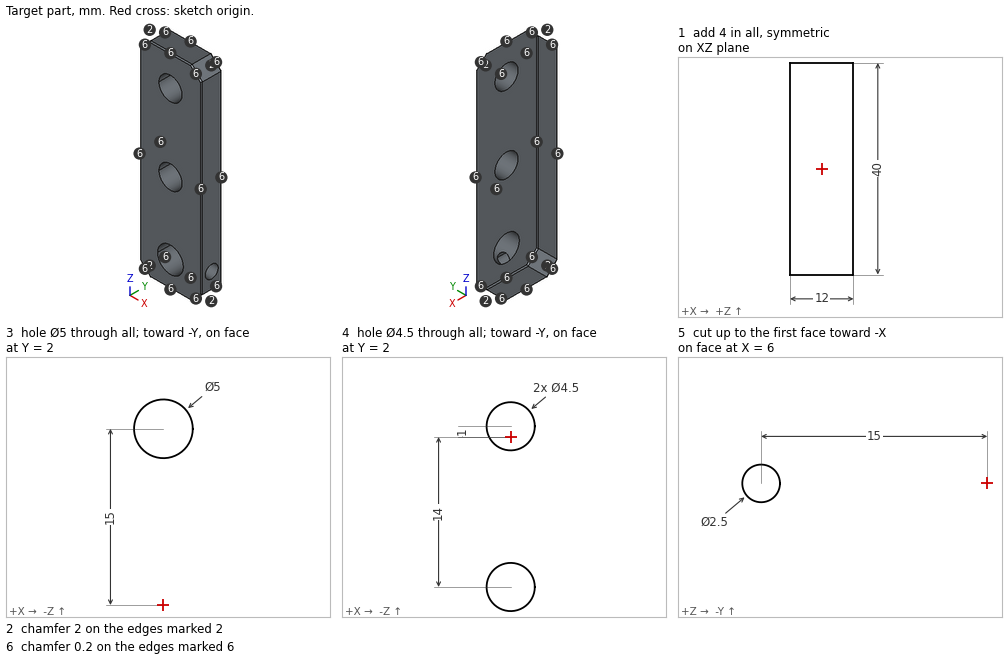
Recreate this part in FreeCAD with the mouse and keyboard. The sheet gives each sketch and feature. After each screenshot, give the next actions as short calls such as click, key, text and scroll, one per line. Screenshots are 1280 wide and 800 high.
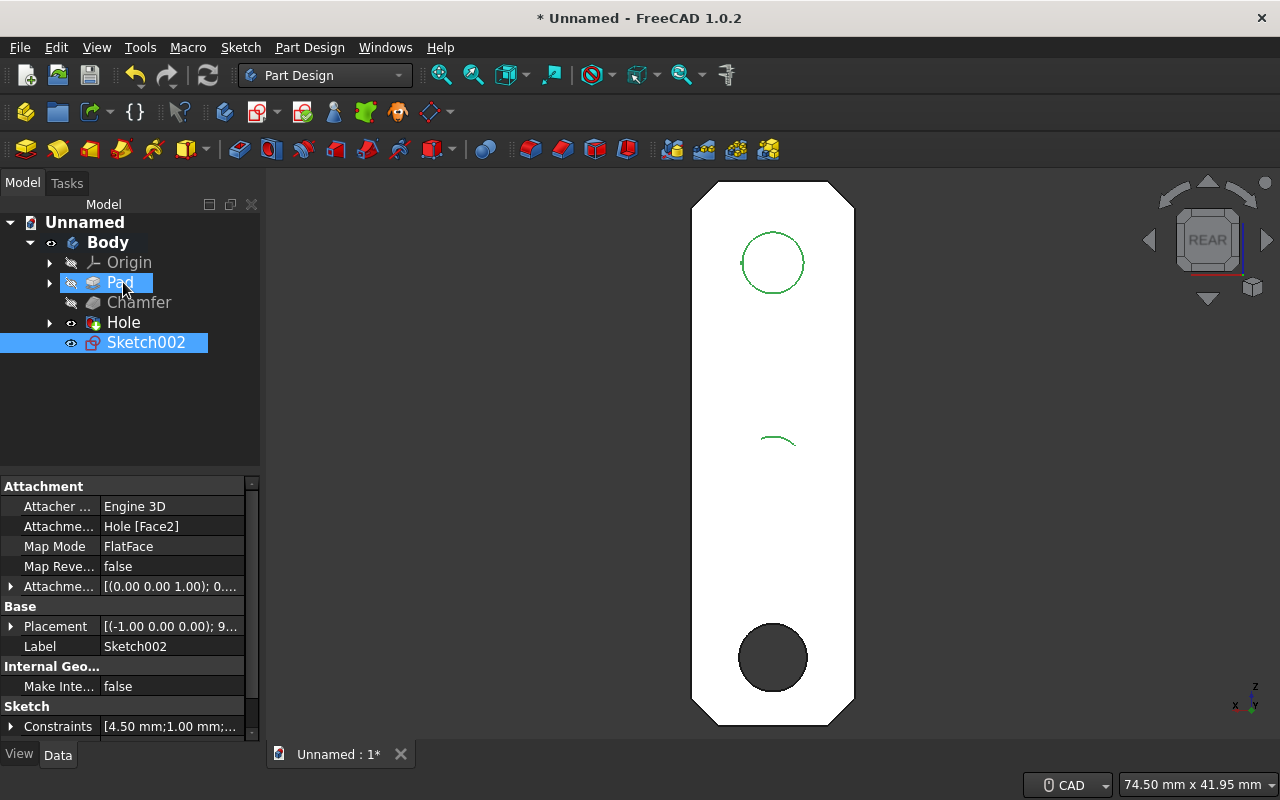
click(272, 150)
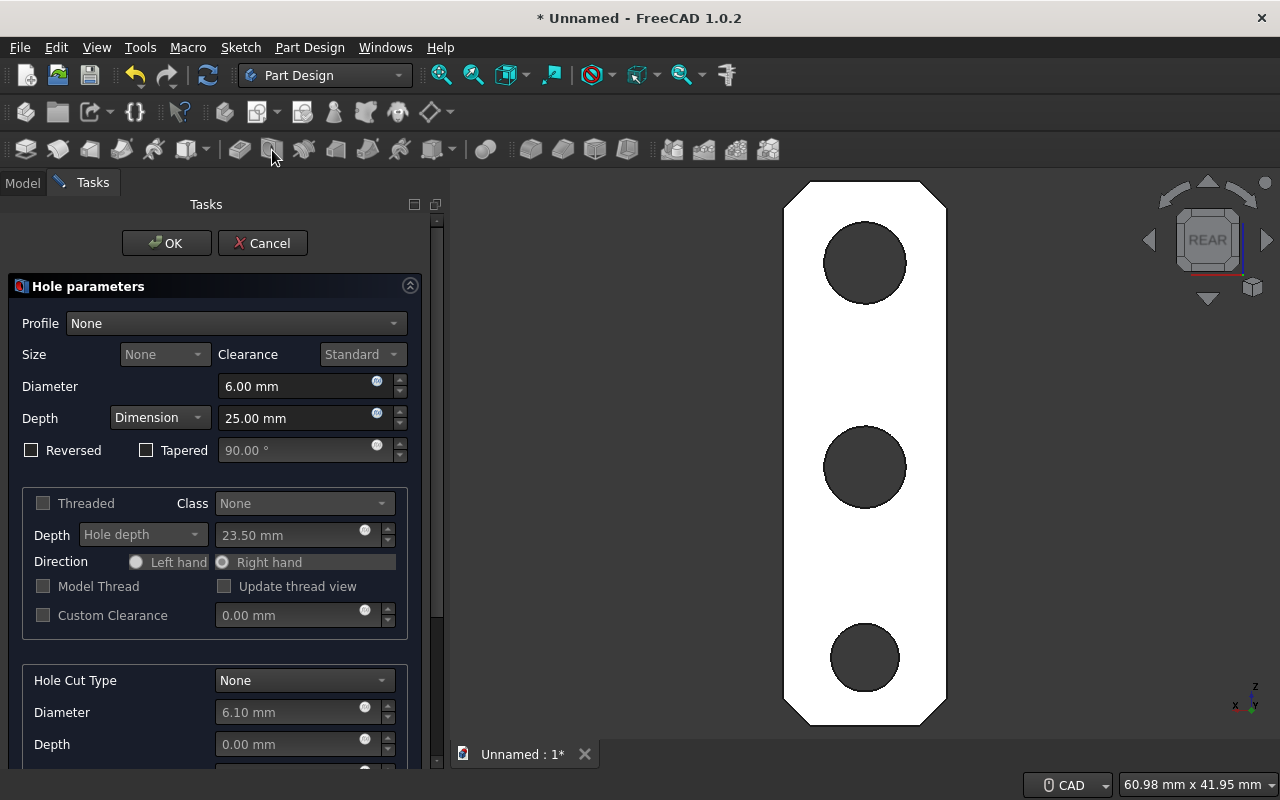
triple_click(305, 386)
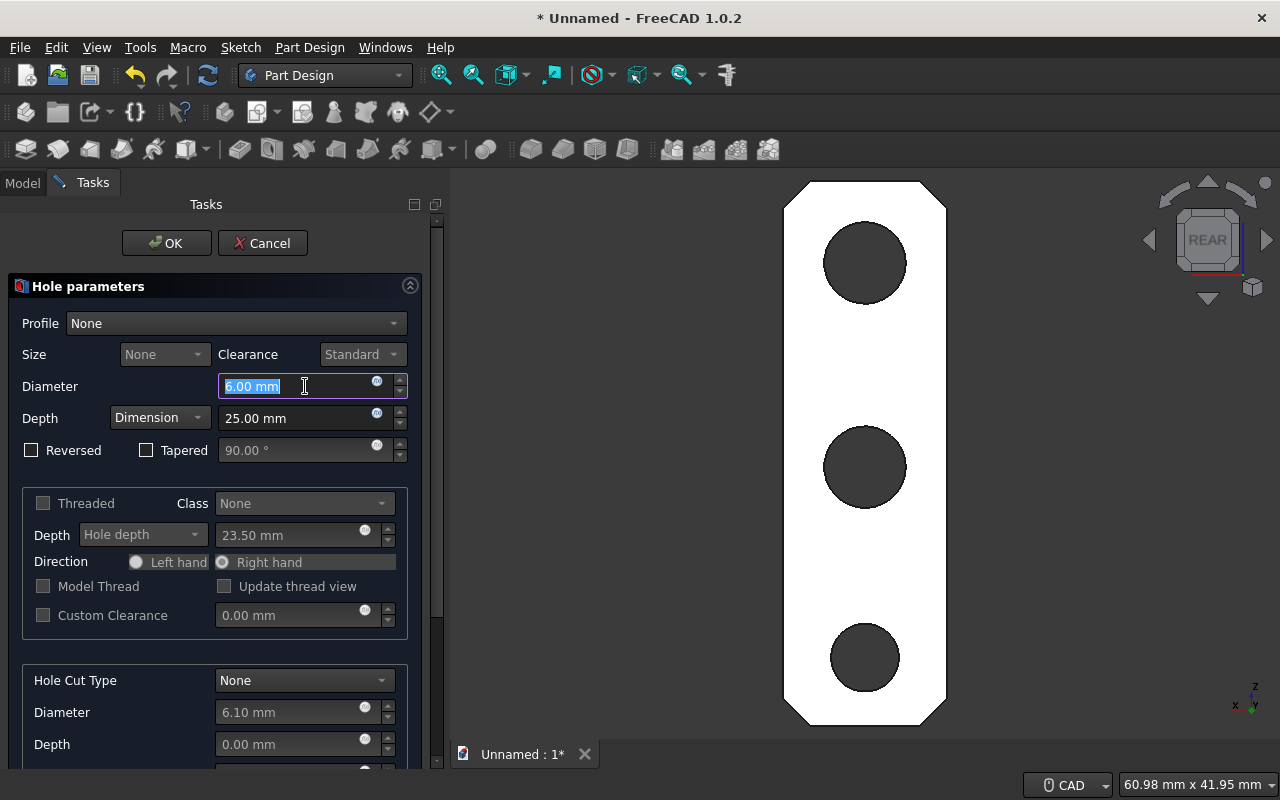
text(4.5)
key(Tab)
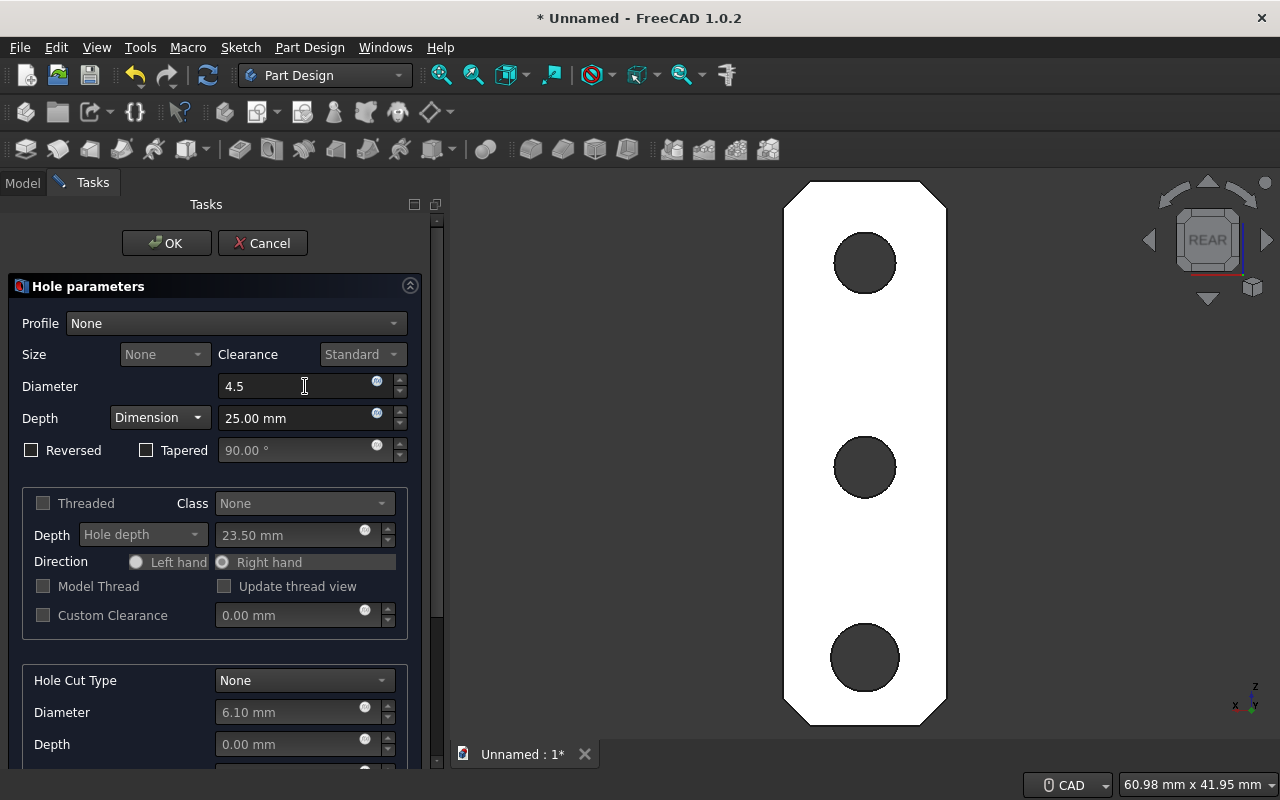
click(161, 418)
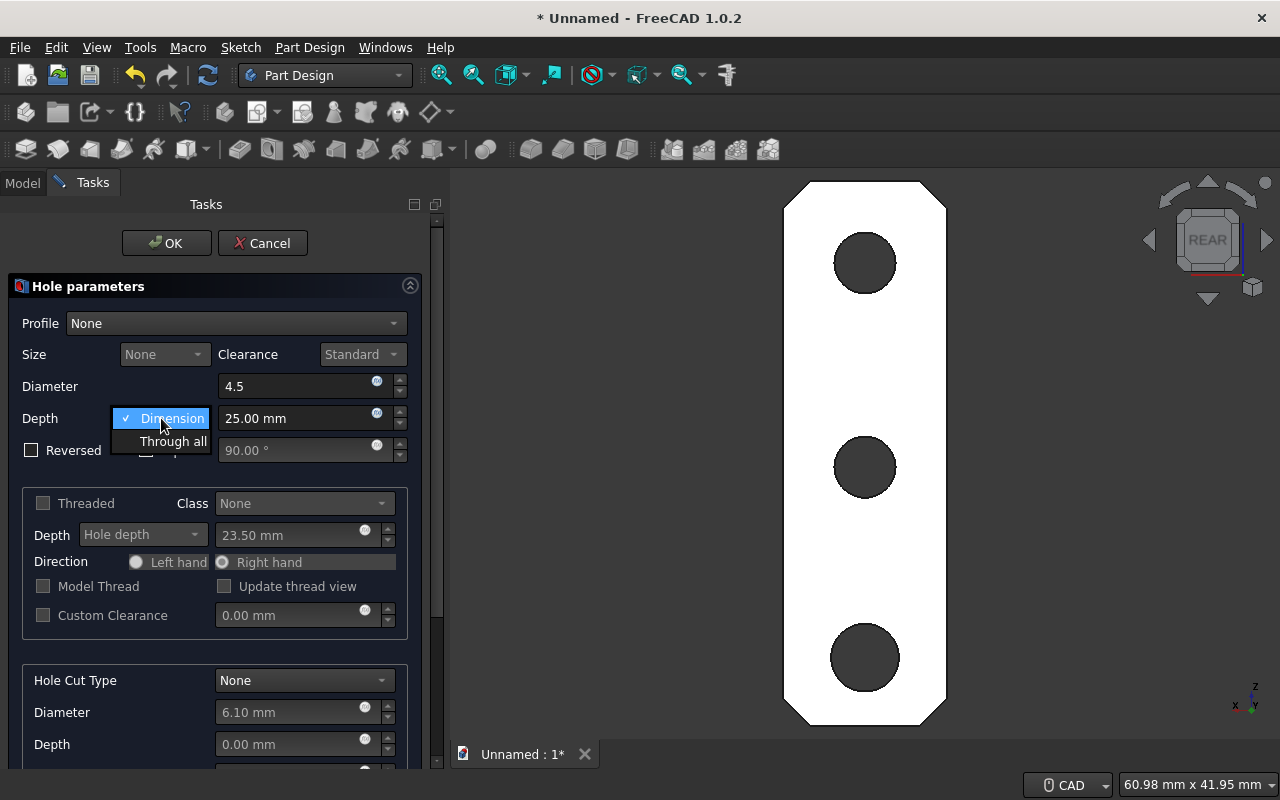
click(160, 442)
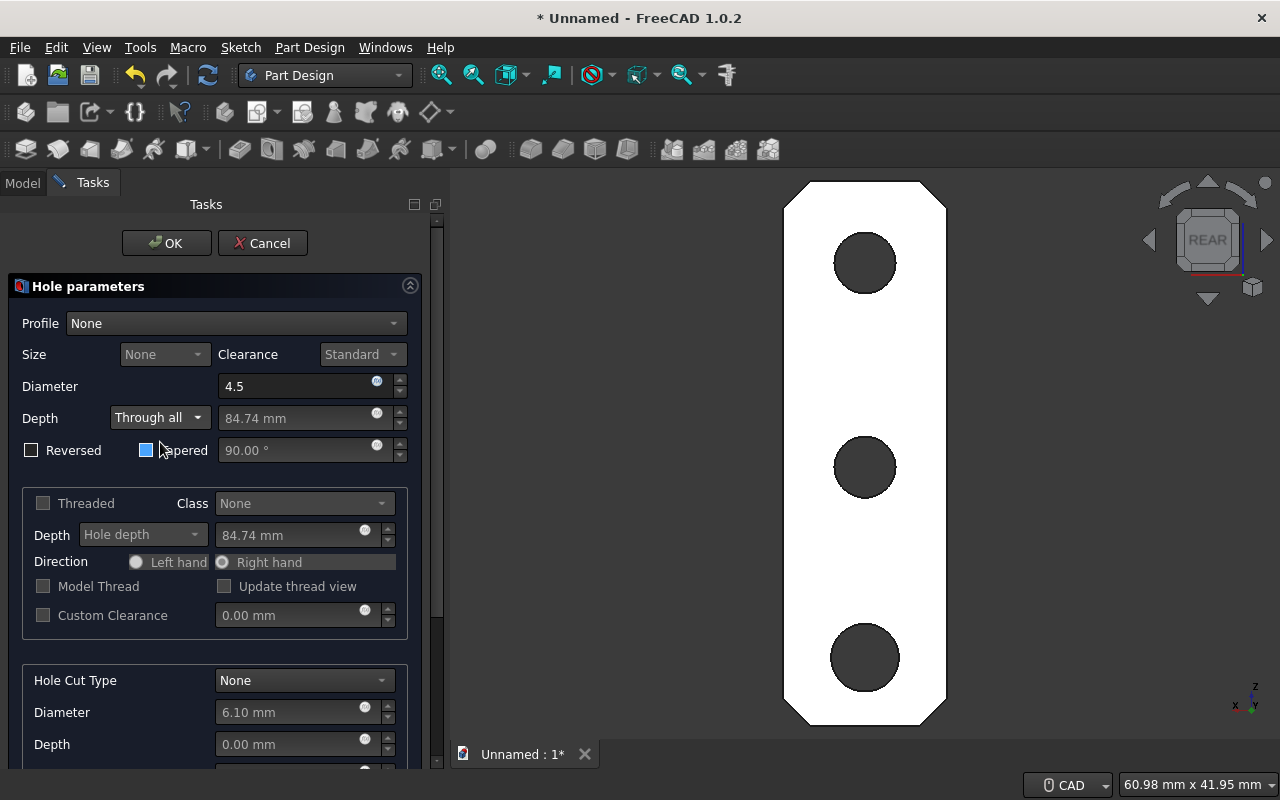
click(167, 243)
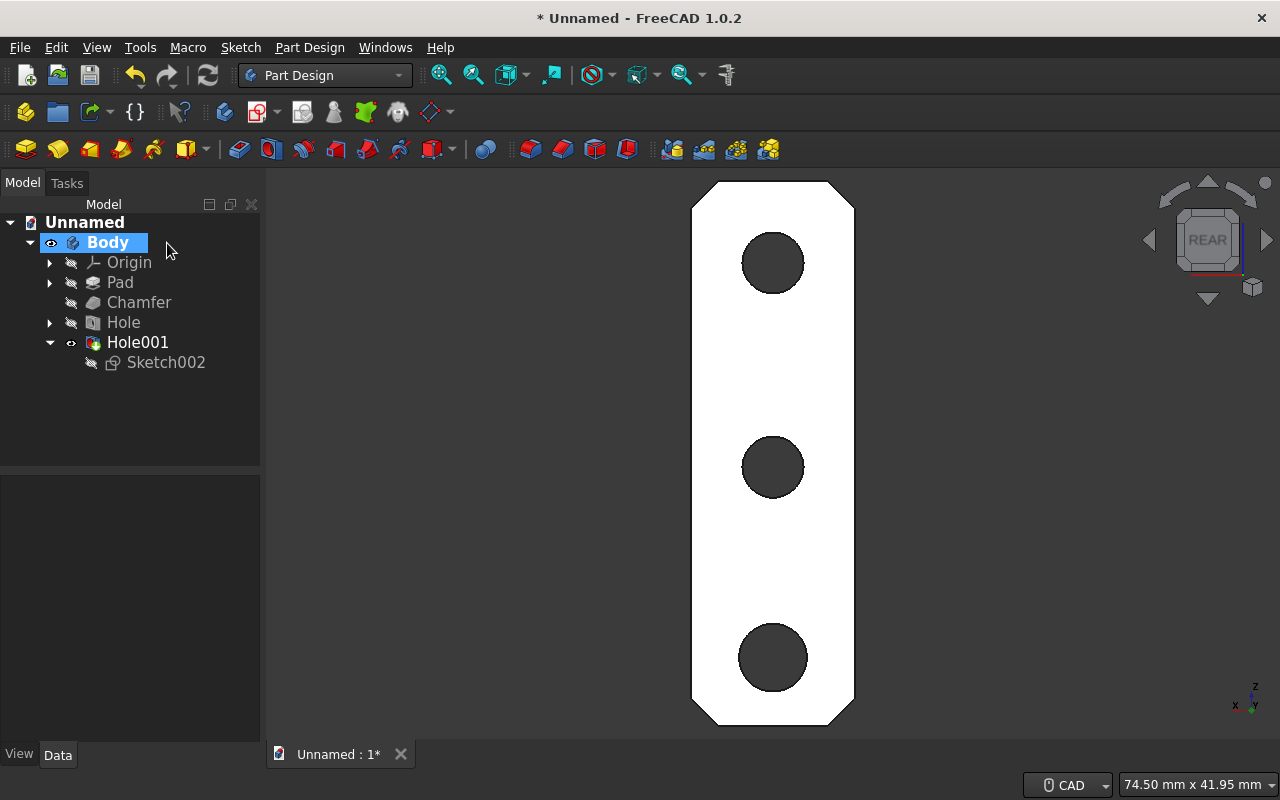
key(0)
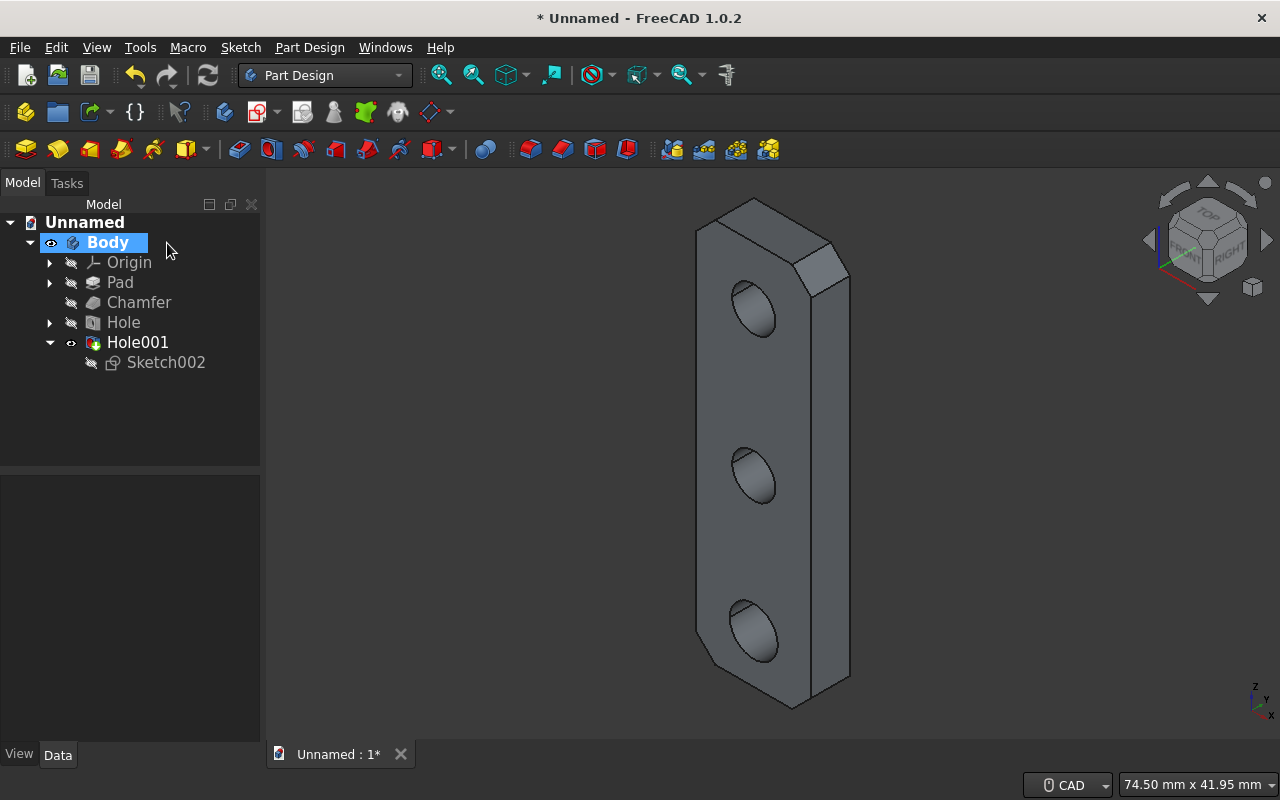
click(831, 314)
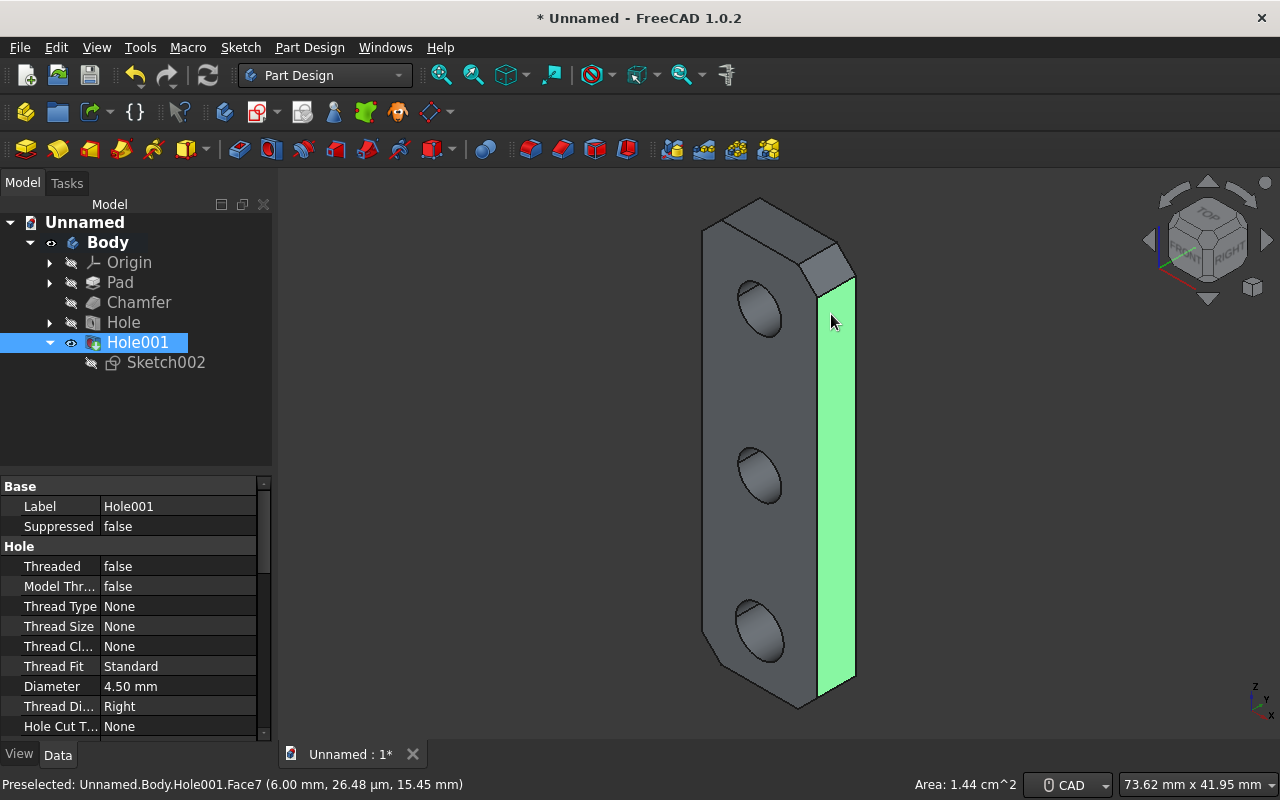
click(258, 112)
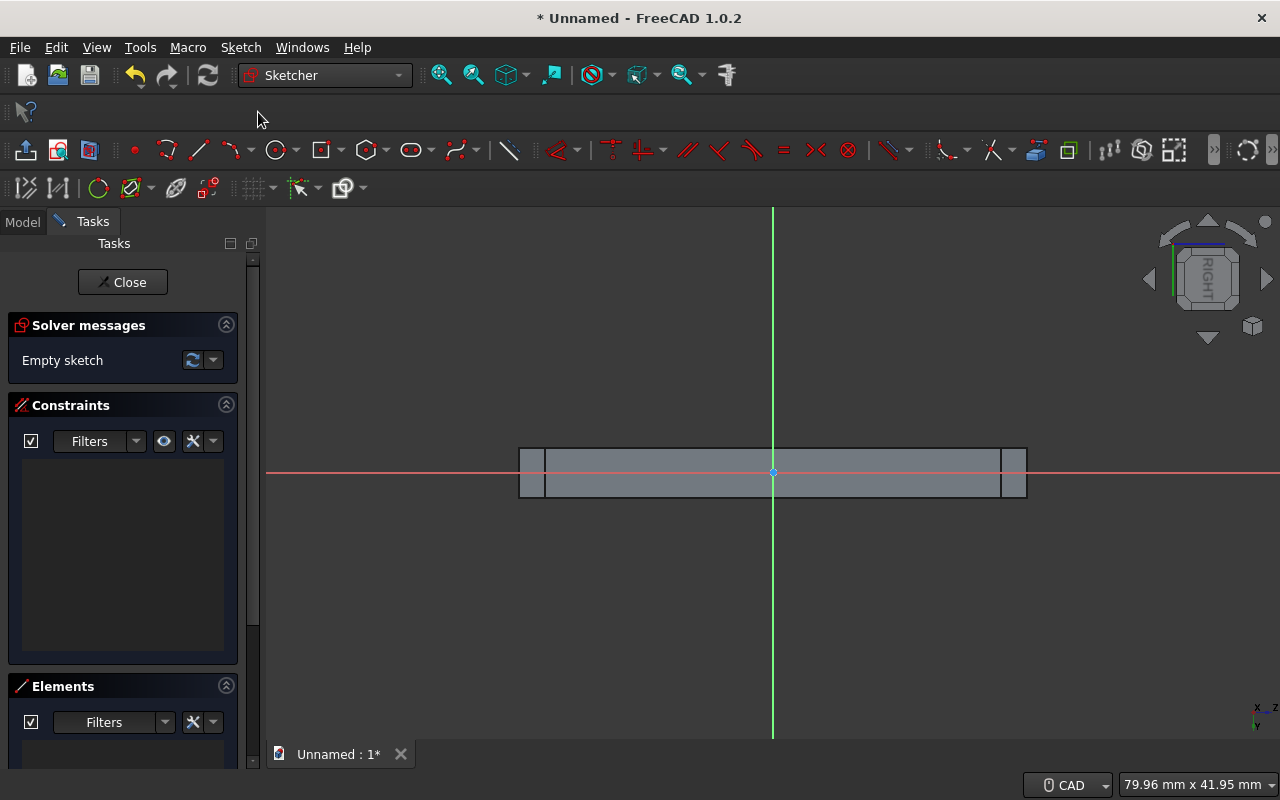
scroll(571, 473, up, 12)